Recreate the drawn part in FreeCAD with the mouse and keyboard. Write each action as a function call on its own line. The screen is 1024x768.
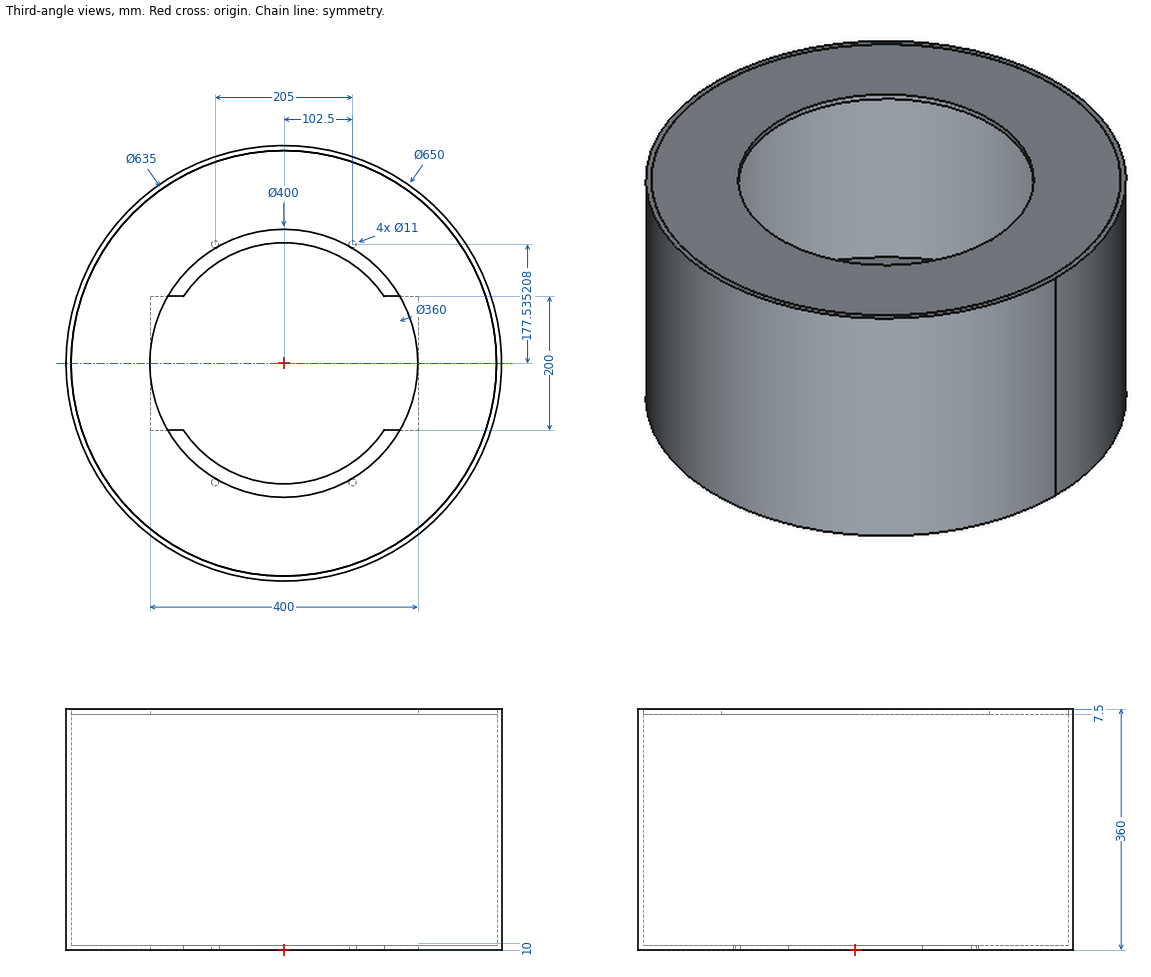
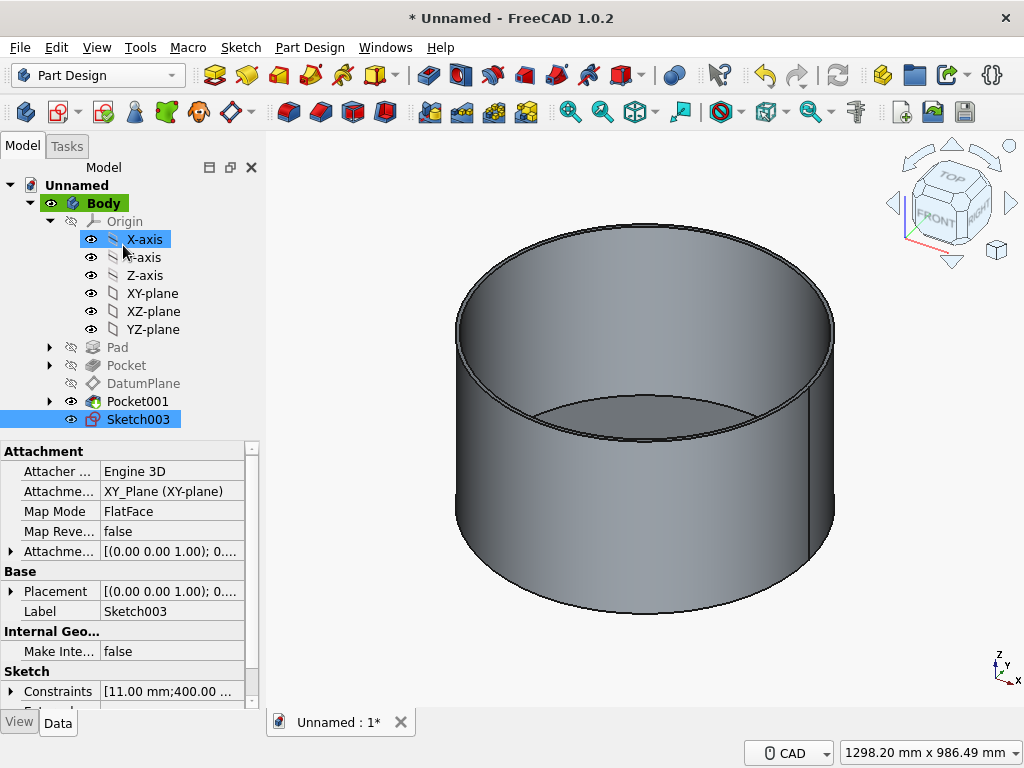
click(430, 76)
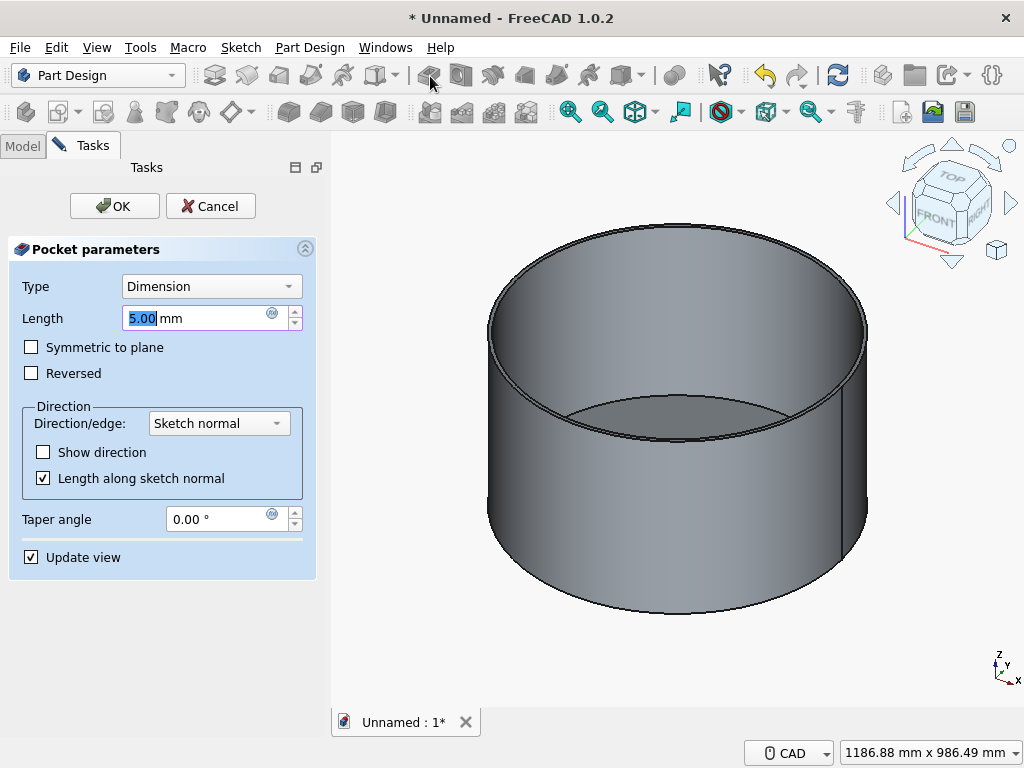
text(10)
key(Tab)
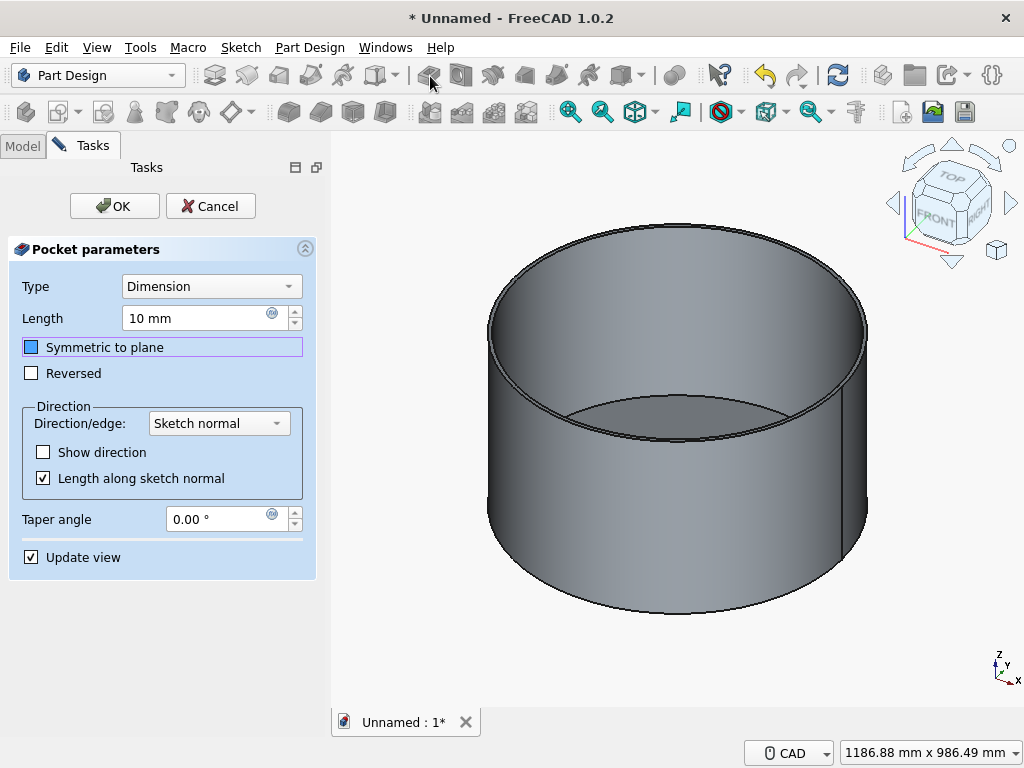
click(30, 373)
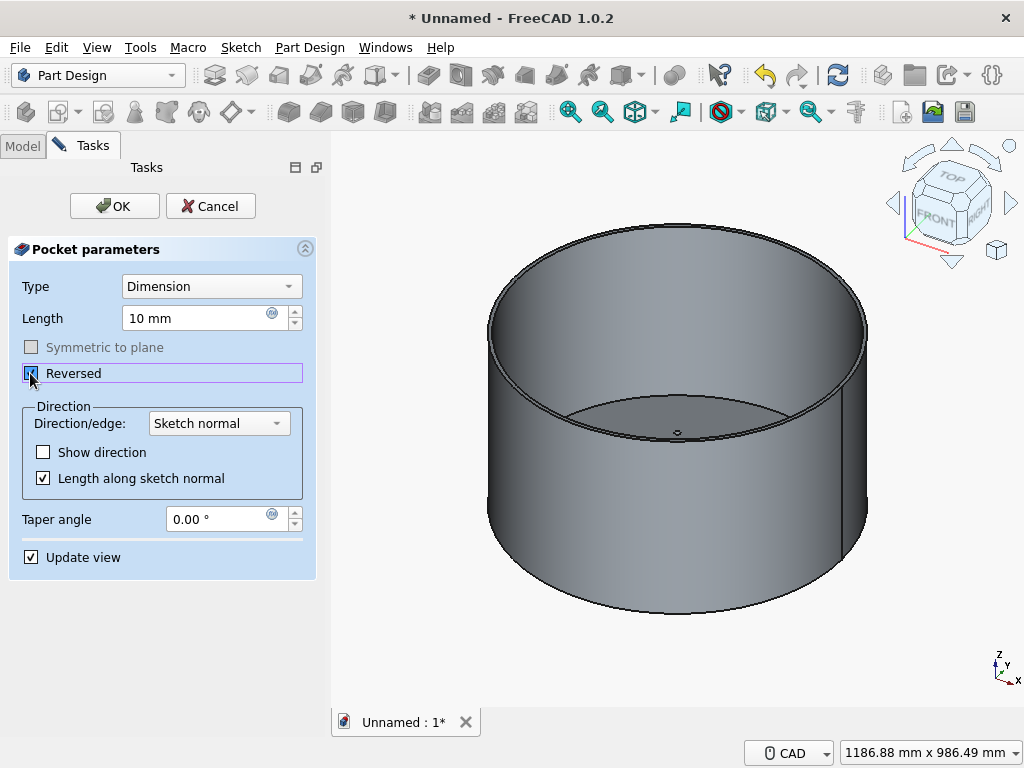
click(115, 206)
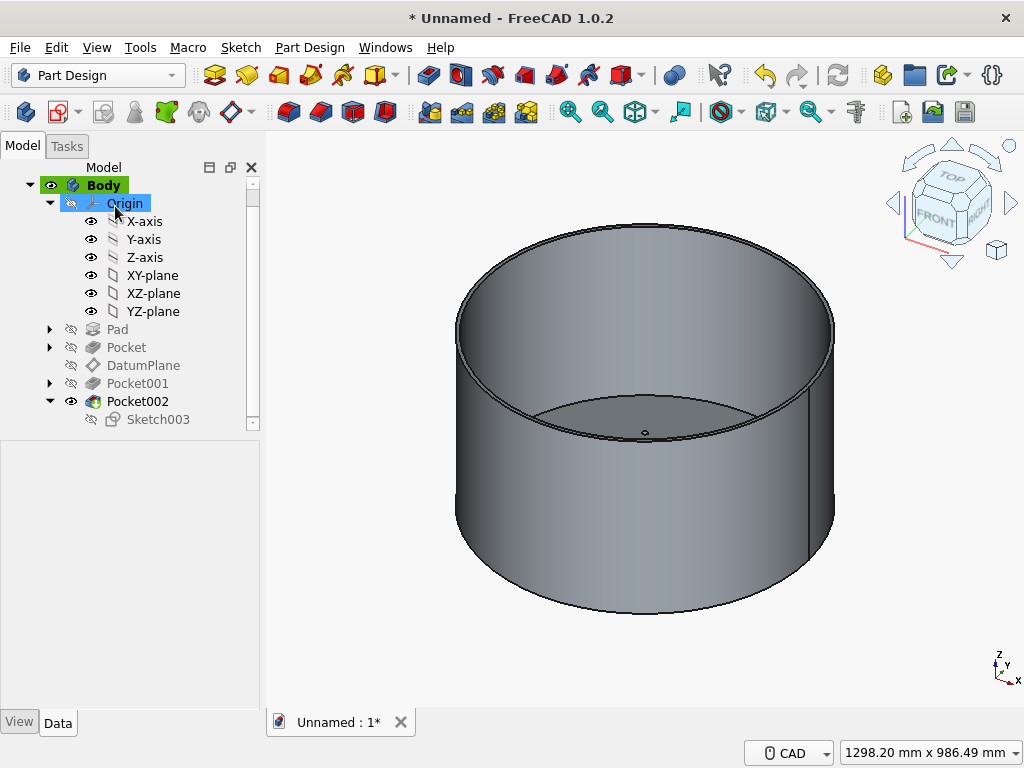
click(26, 112)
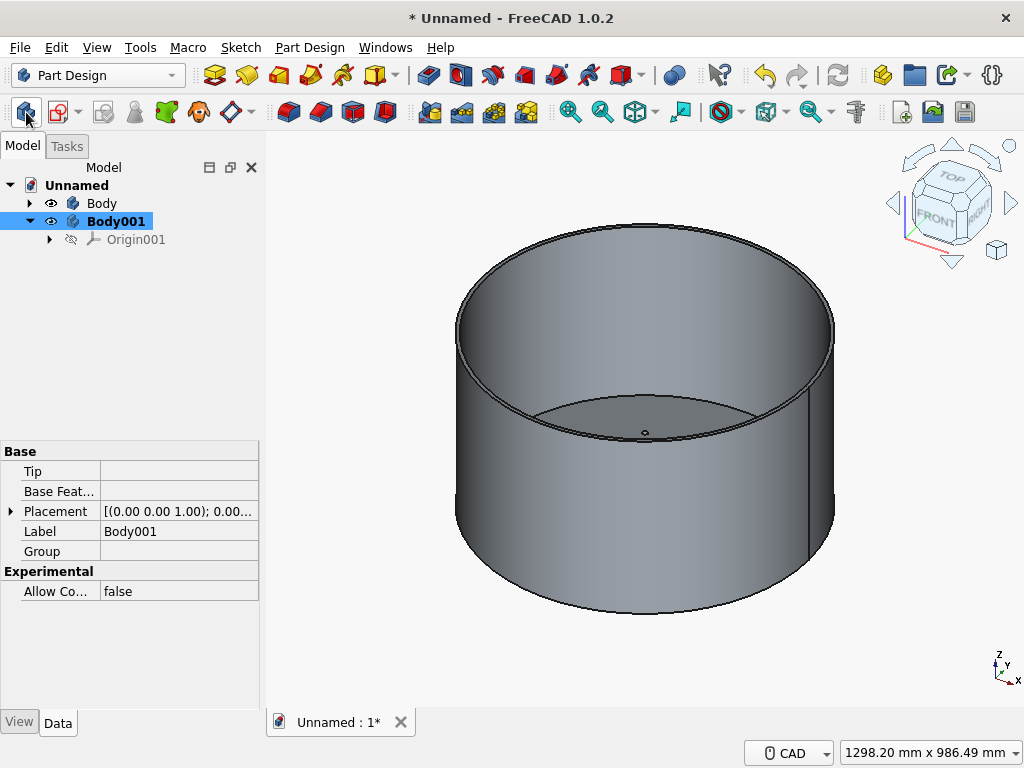
click(50, 239)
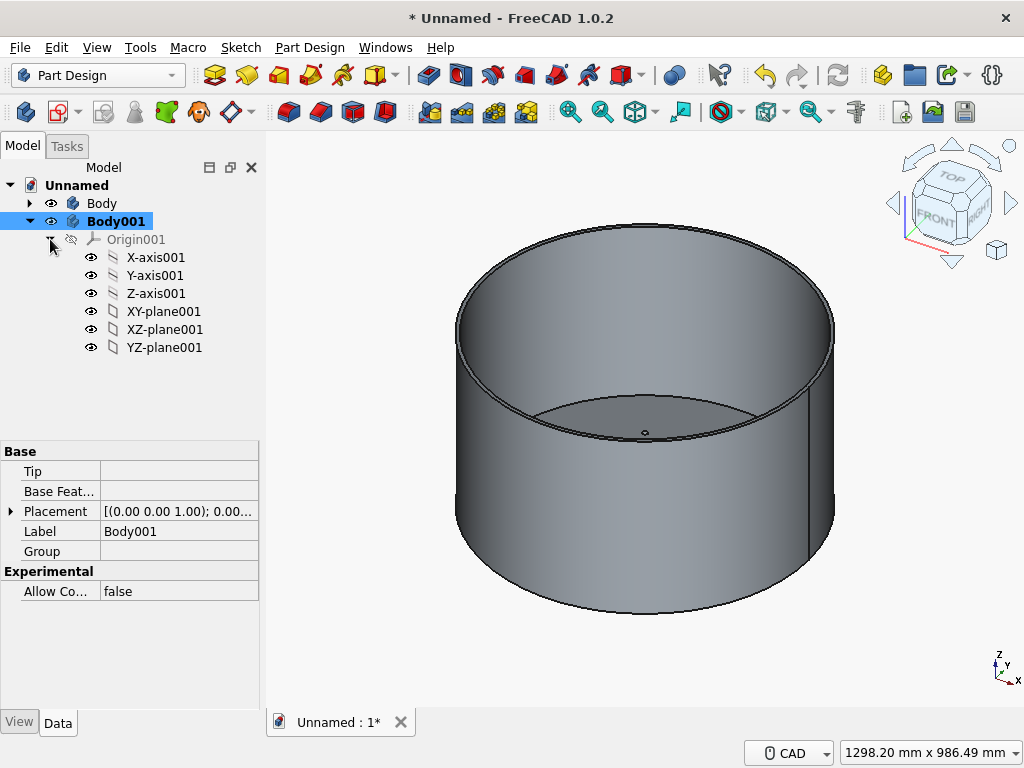
click(136, 311)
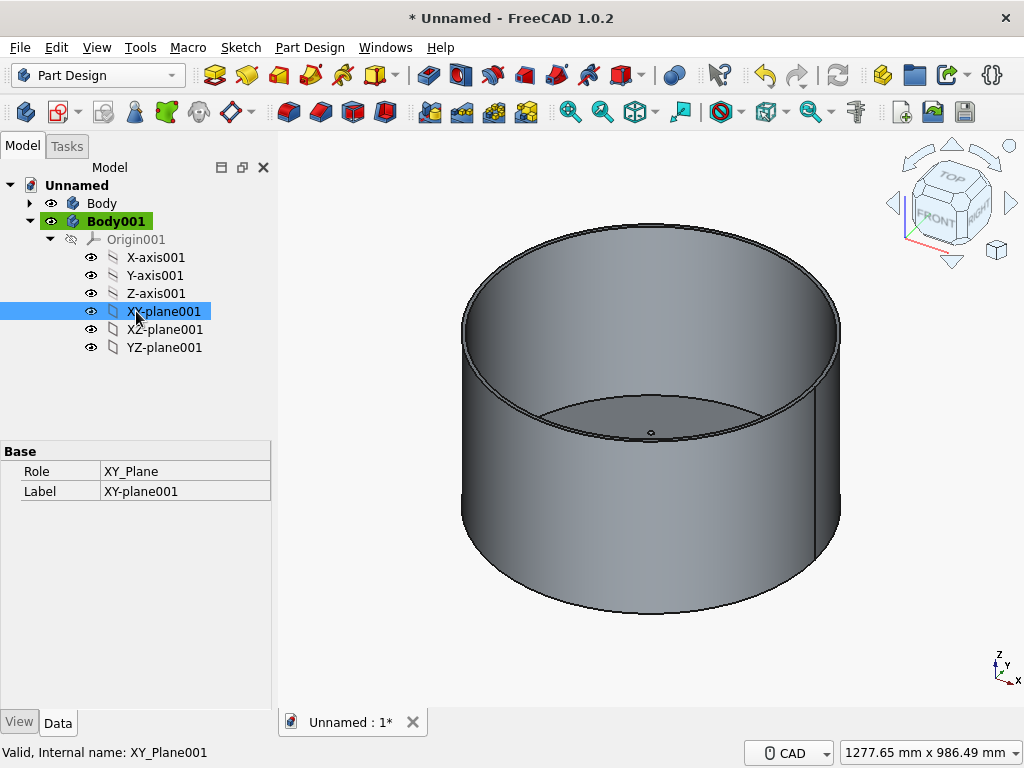
click(232, 112)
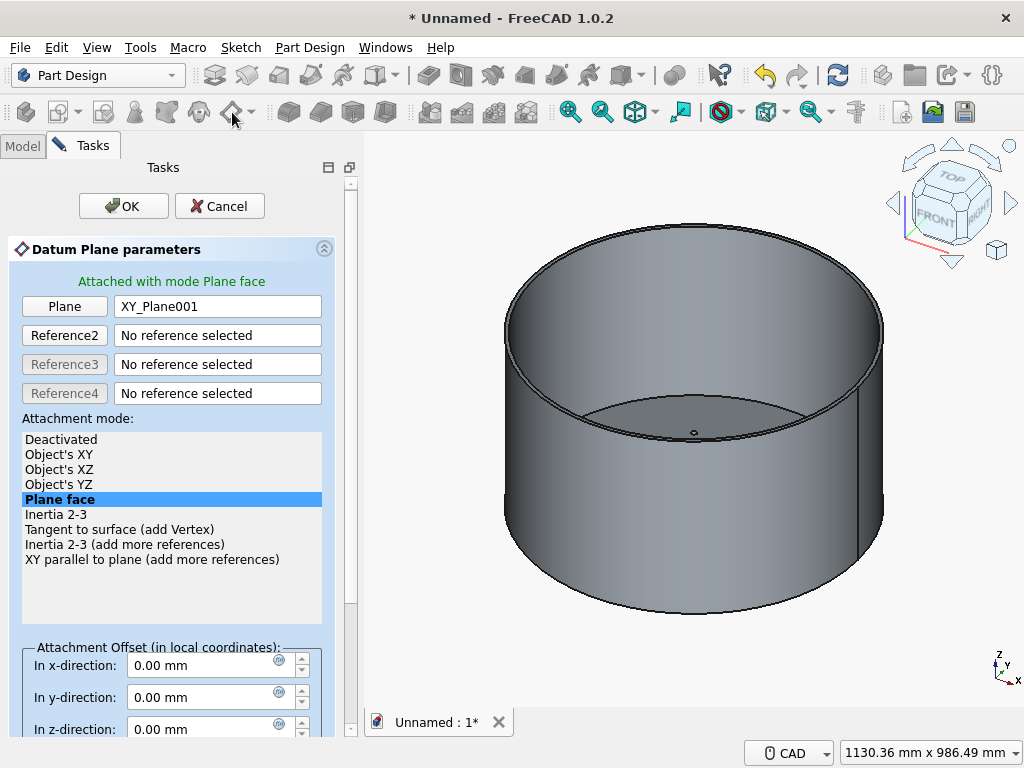
scroll(351, 456, down, 2)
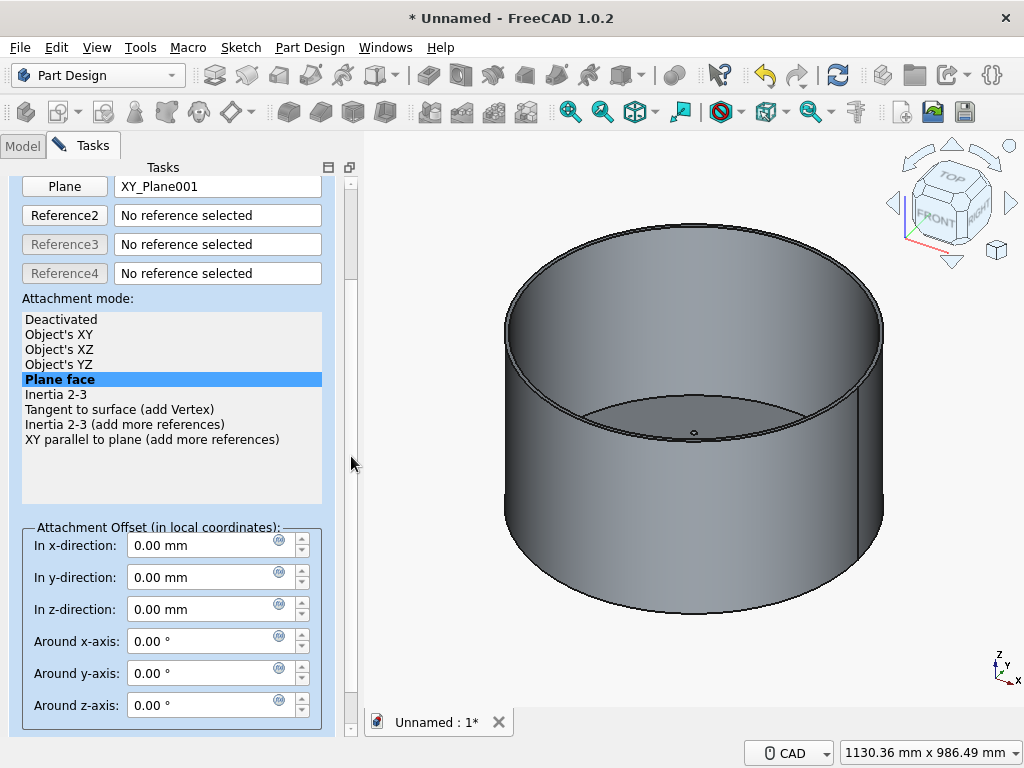
triple_click(210, 609)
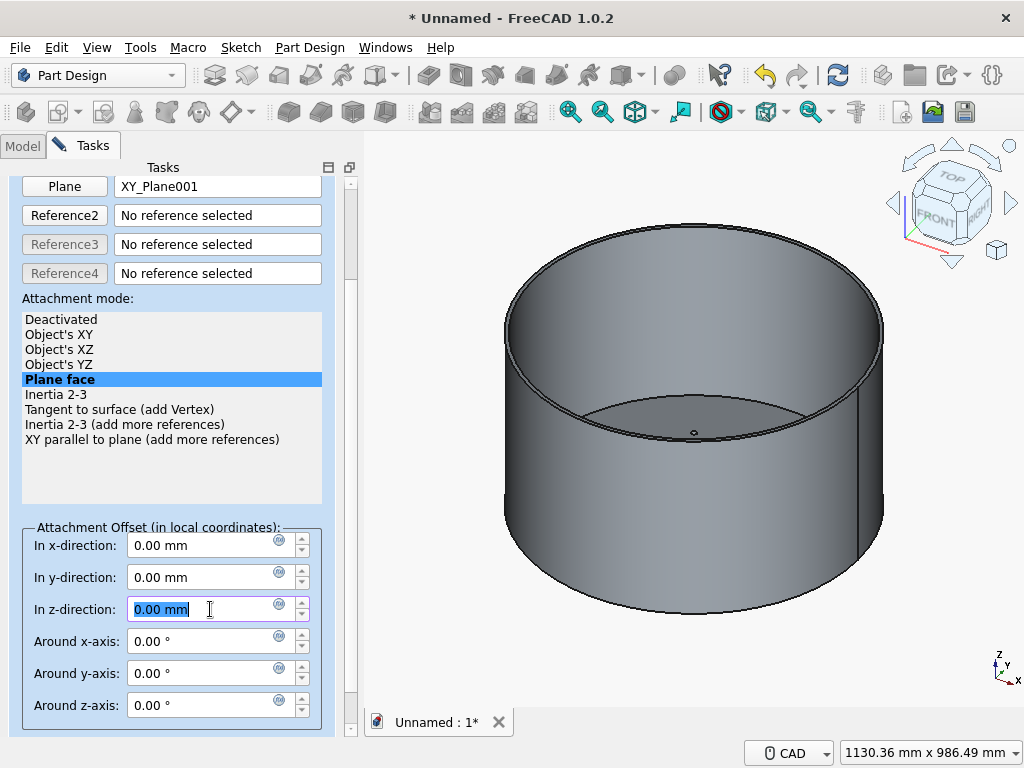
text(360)
key(Tab)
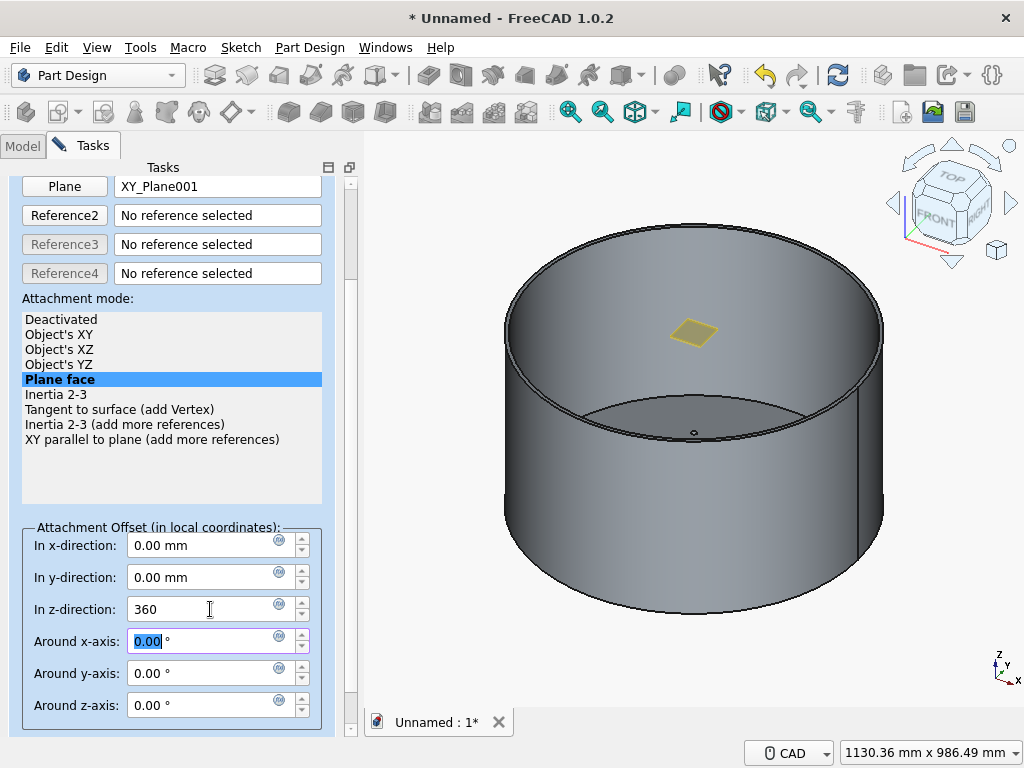
scroll(351, 456, up, 3)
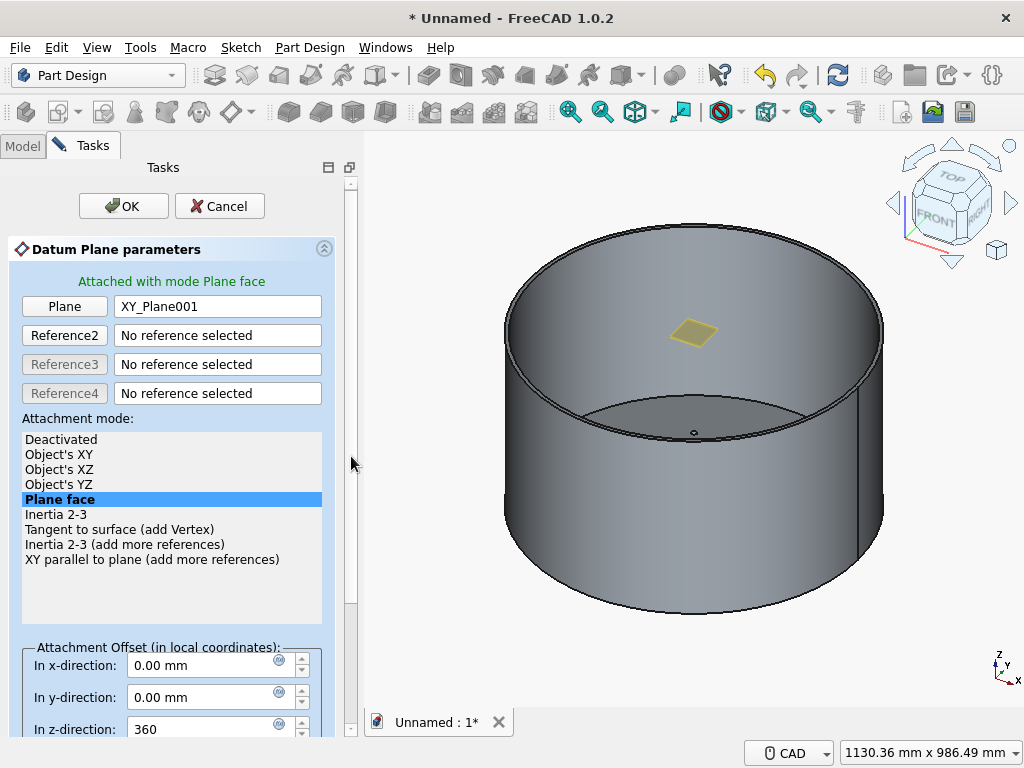
click(124, 206)